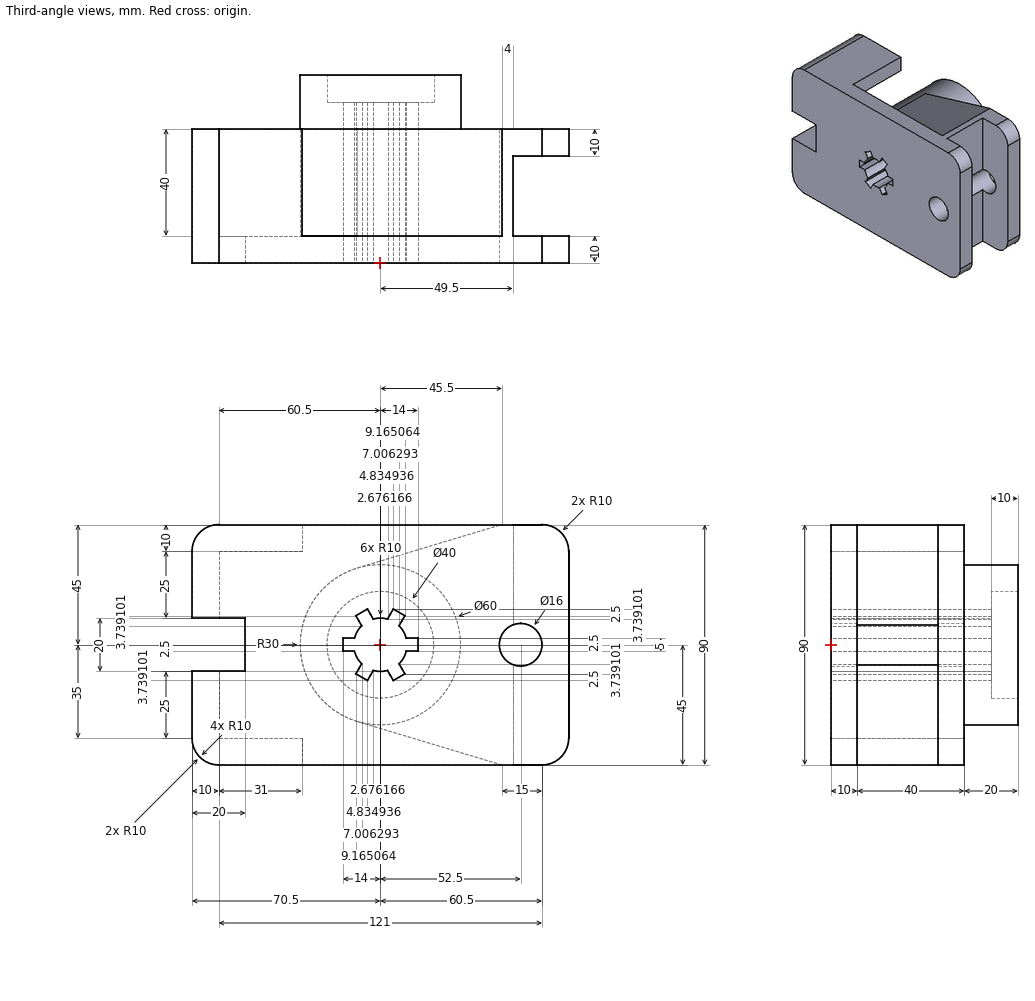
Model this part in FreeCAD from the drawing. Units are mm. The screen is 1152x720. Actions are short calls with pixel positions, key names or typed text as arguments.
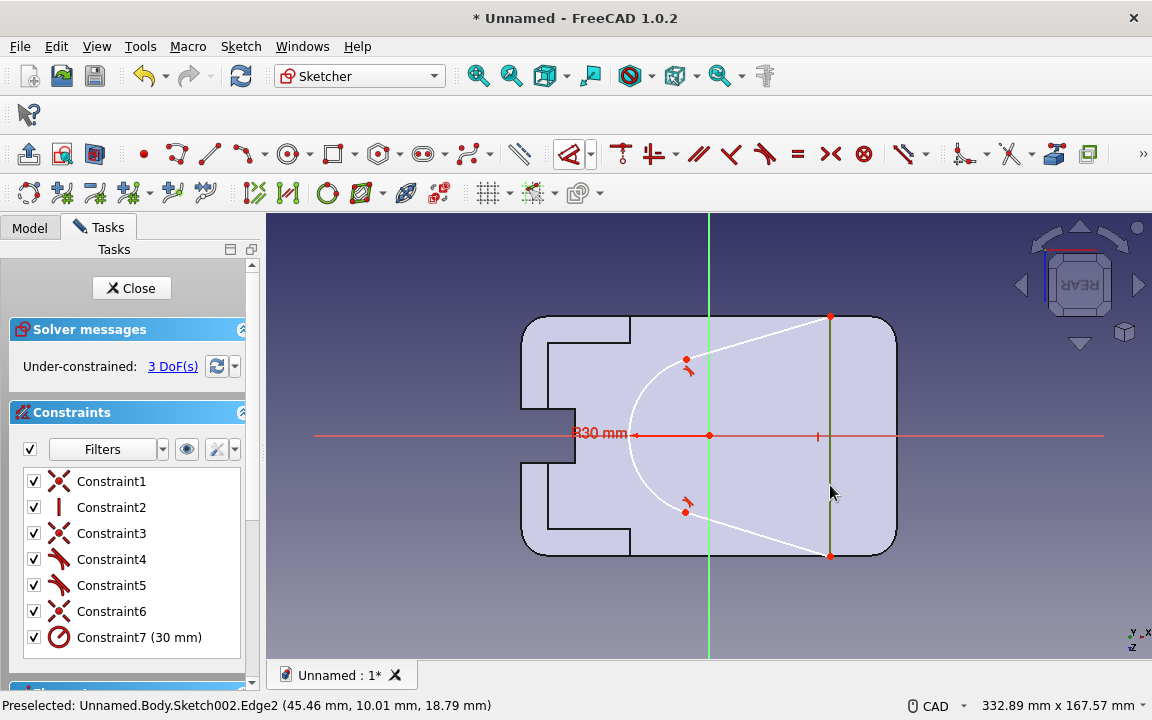
key(i)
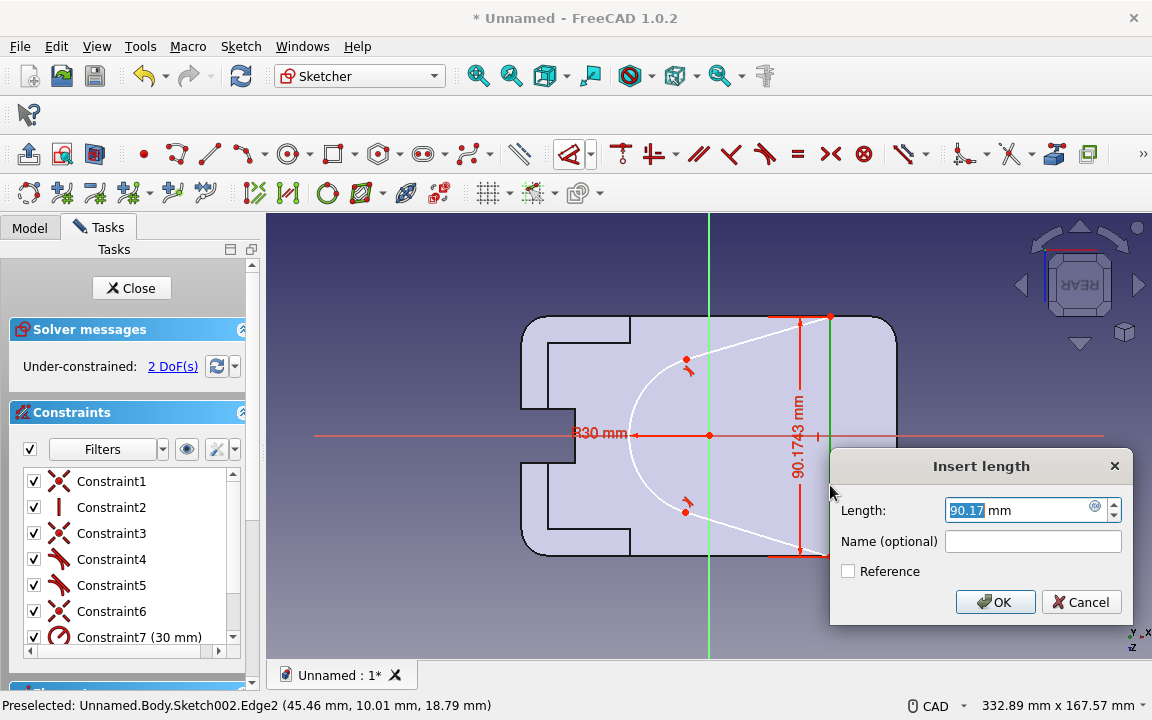
text(90)
key(Return)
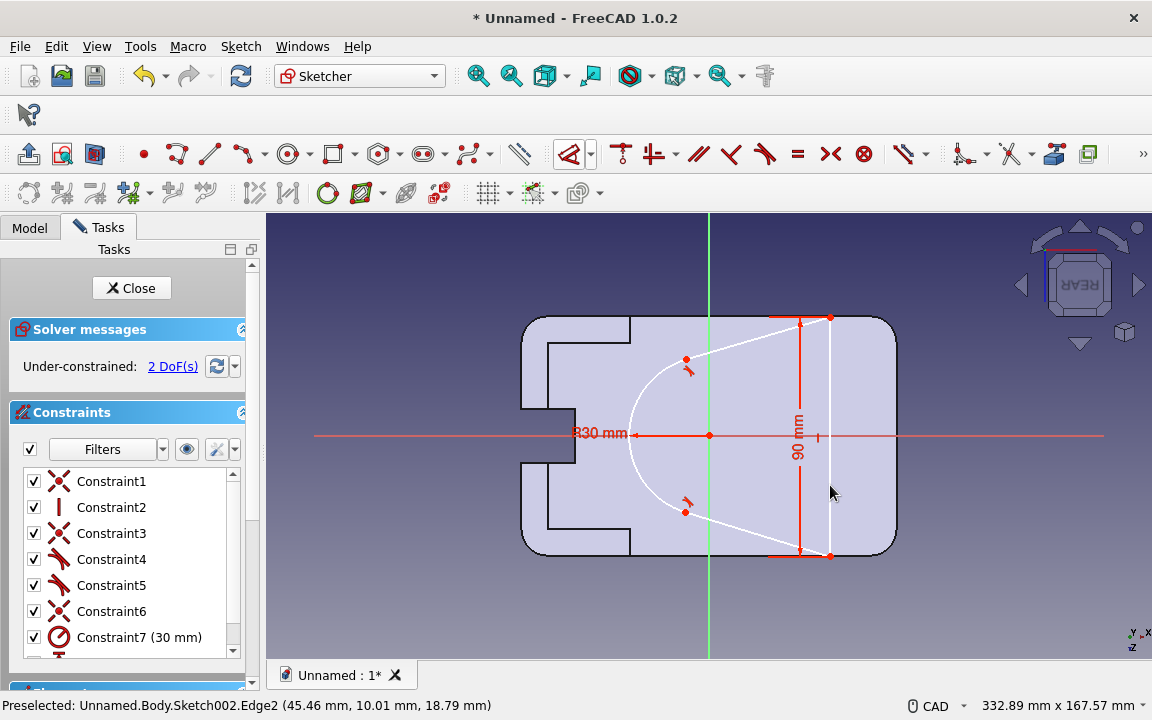
click(830, 557)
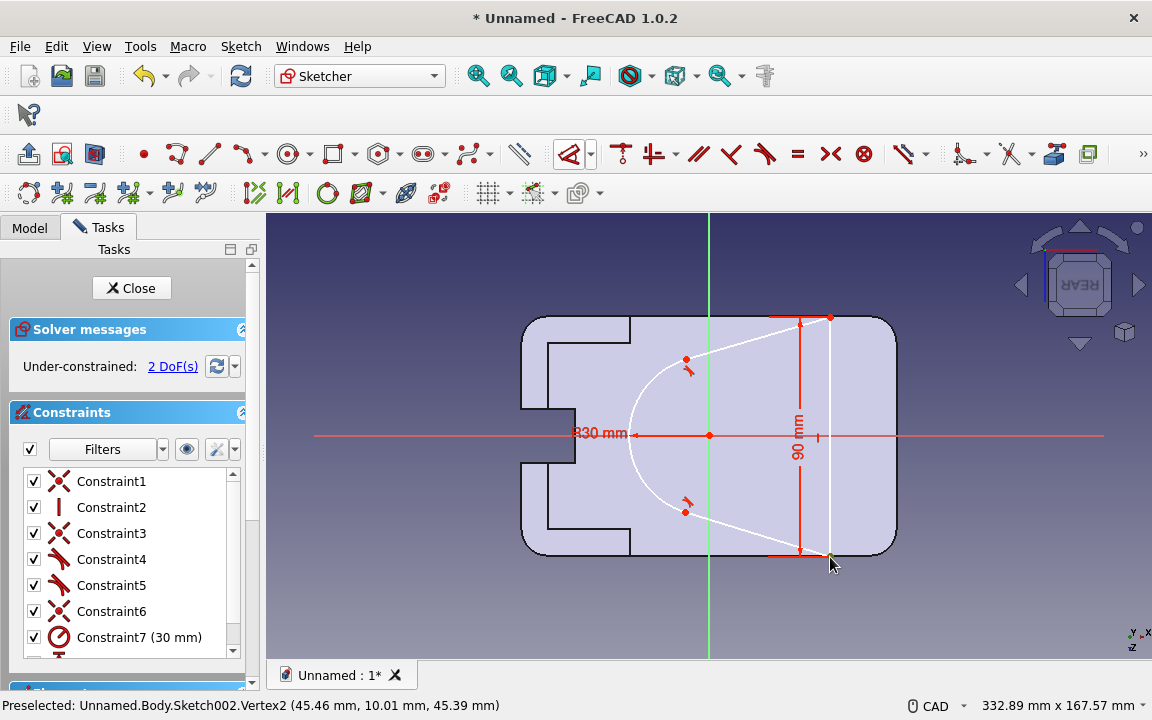
key(i)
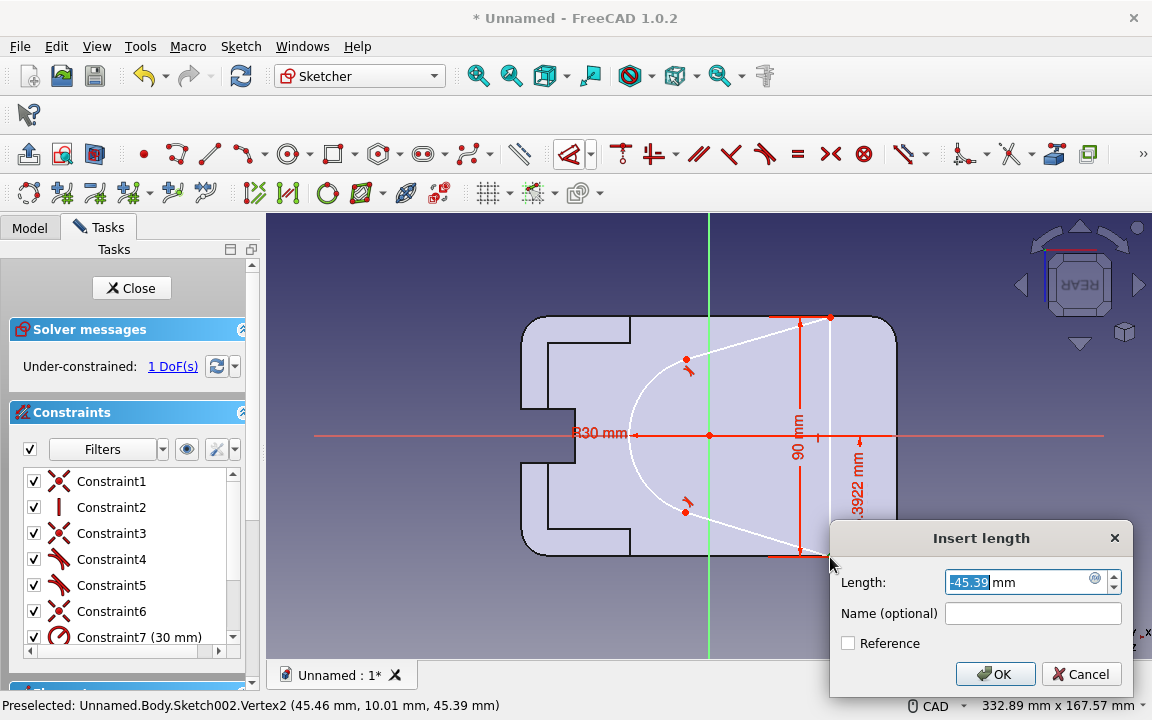
text(-45)
key(Return)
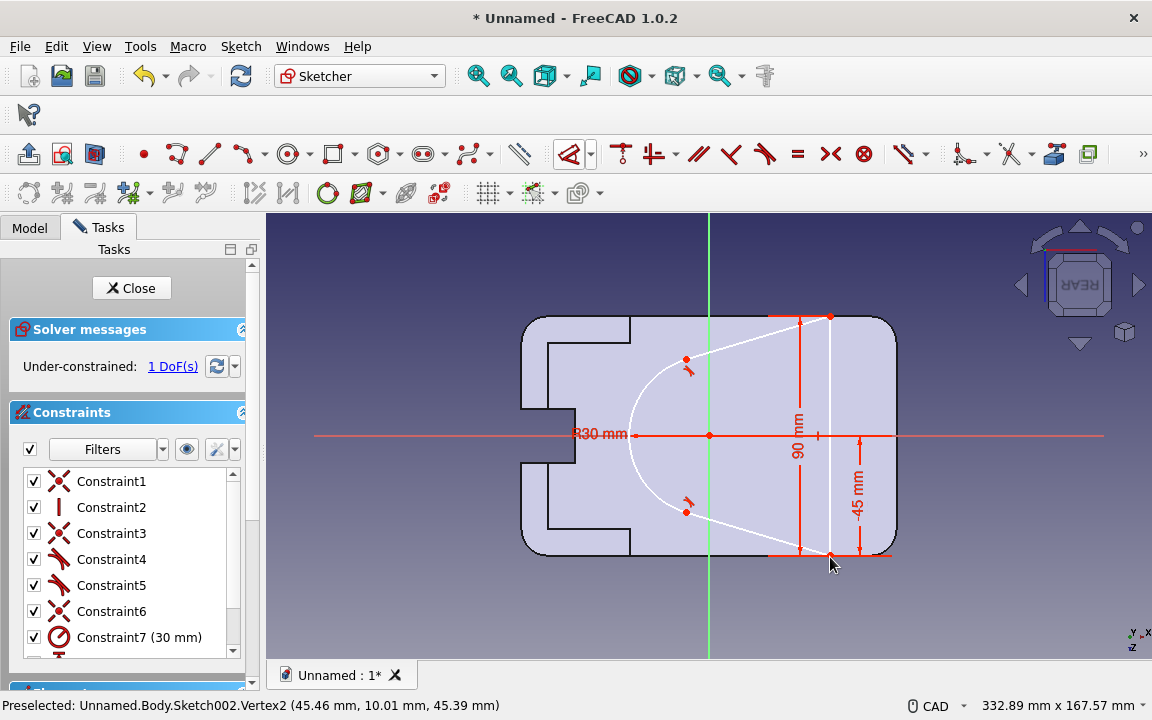
click(830, 556)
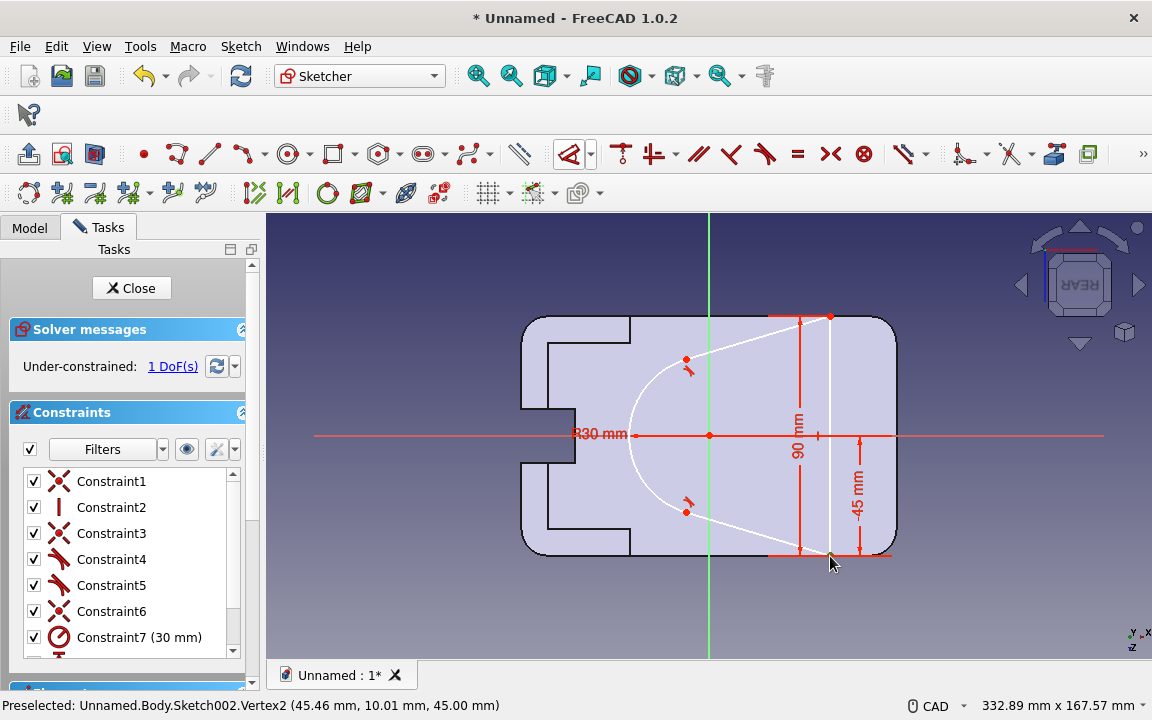
click(590, 154)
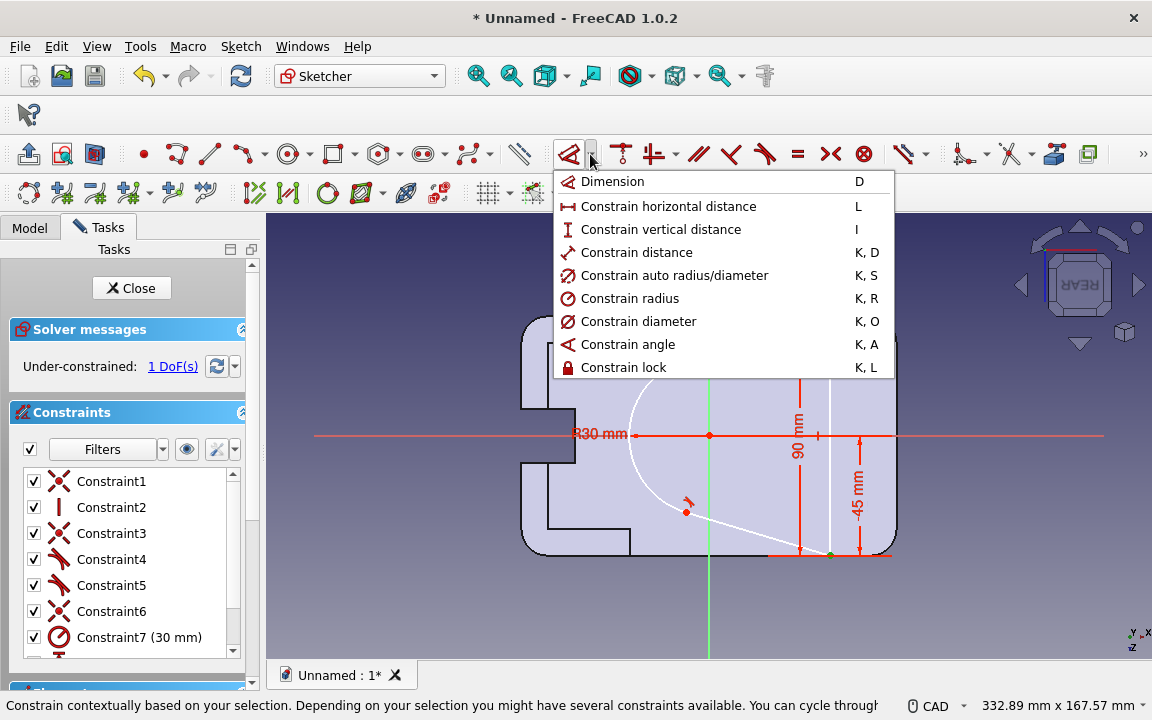
click(724, 206)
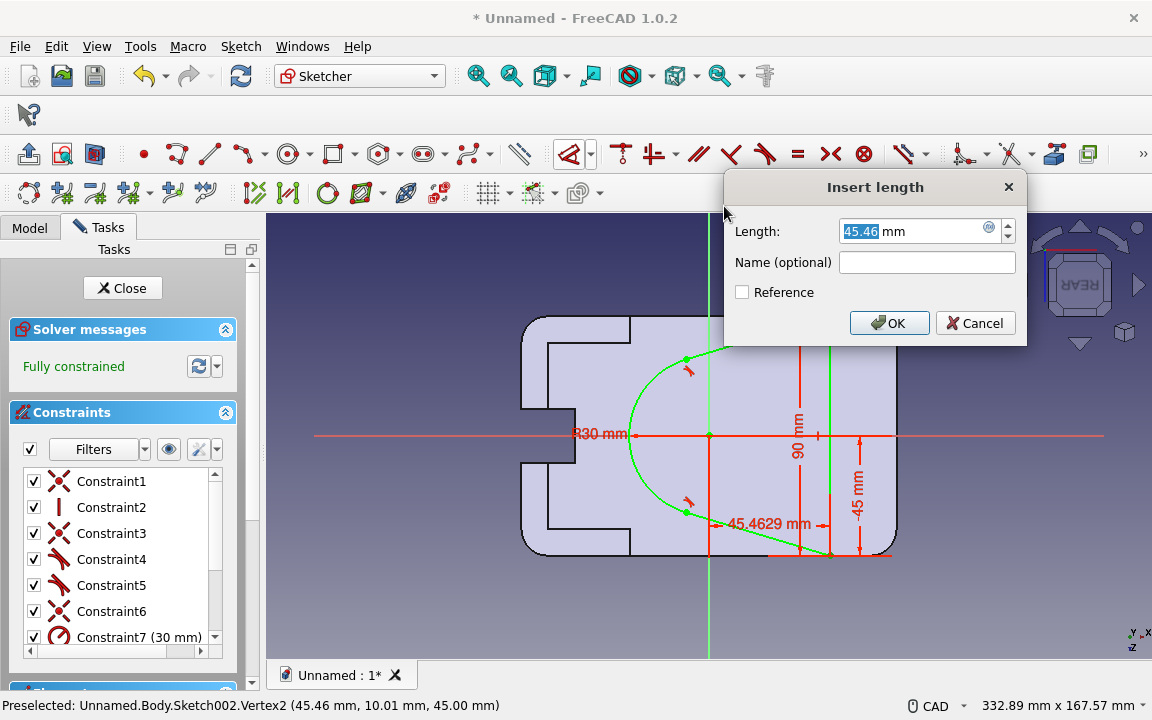
text(45.5)
key(Return)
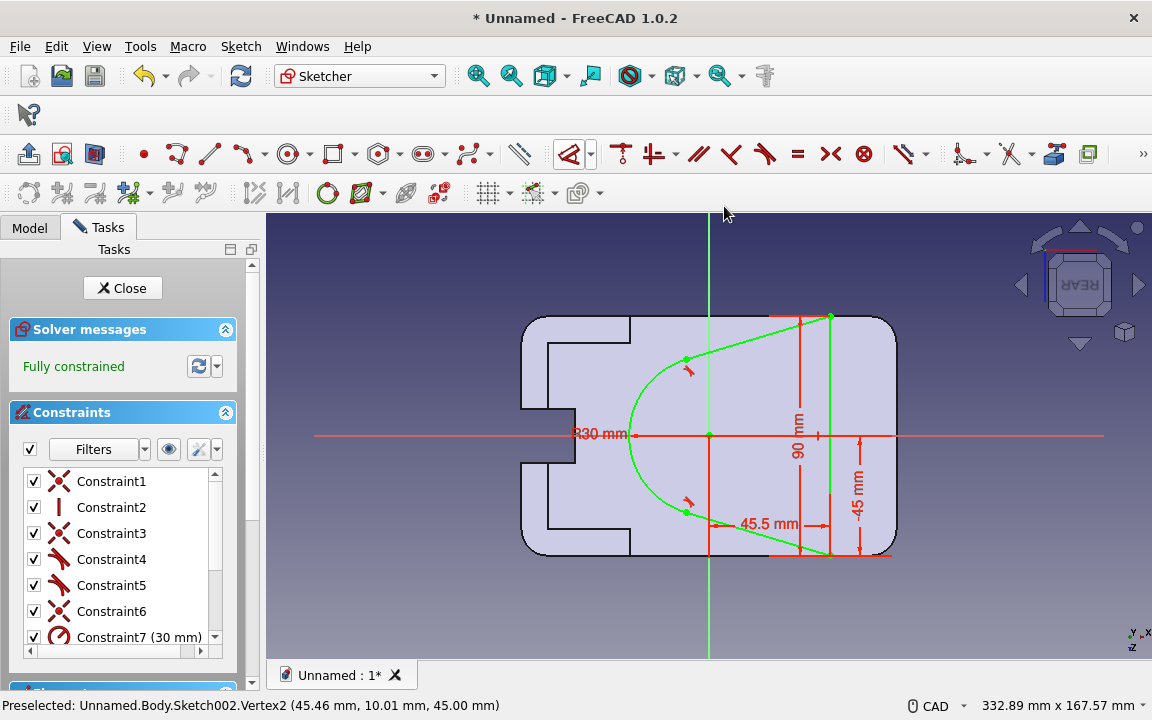
click(123, 288)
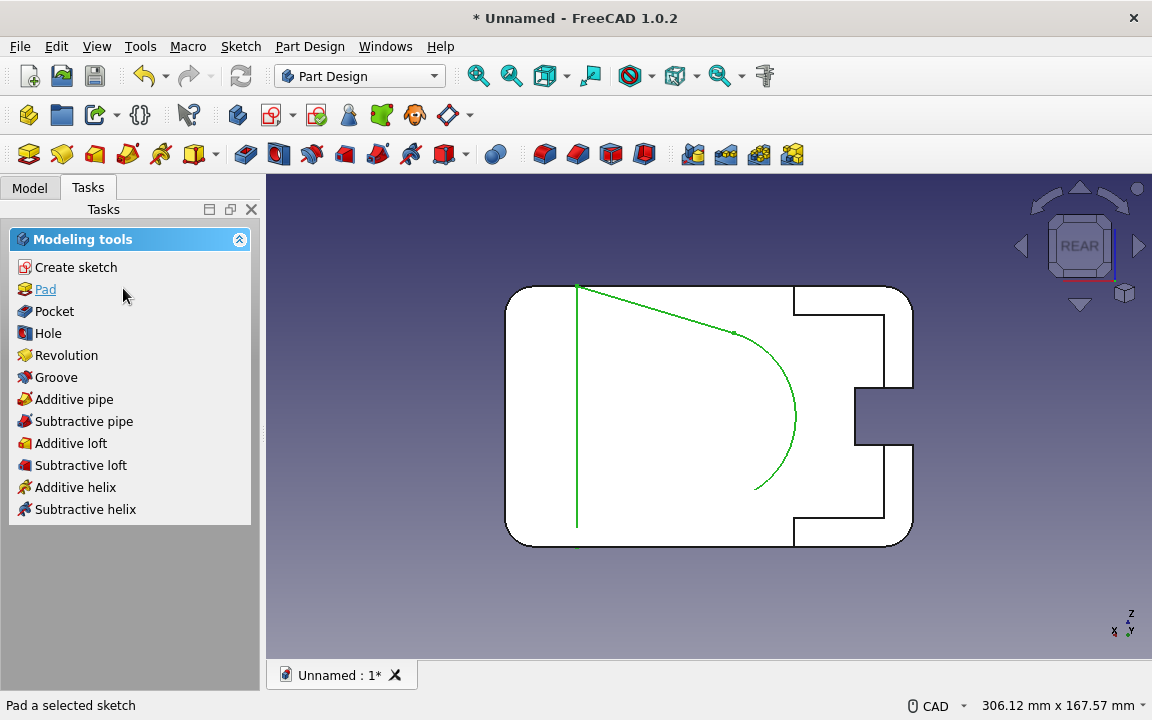
click(29, 154)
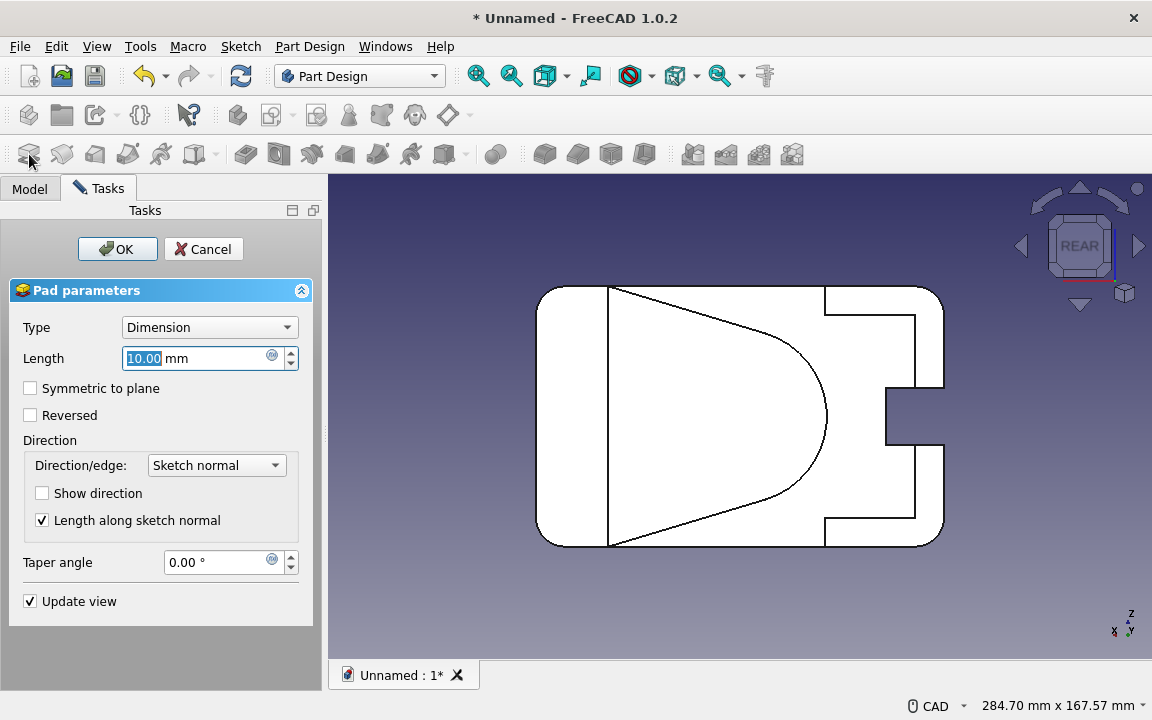
text(40)
key(Tab)